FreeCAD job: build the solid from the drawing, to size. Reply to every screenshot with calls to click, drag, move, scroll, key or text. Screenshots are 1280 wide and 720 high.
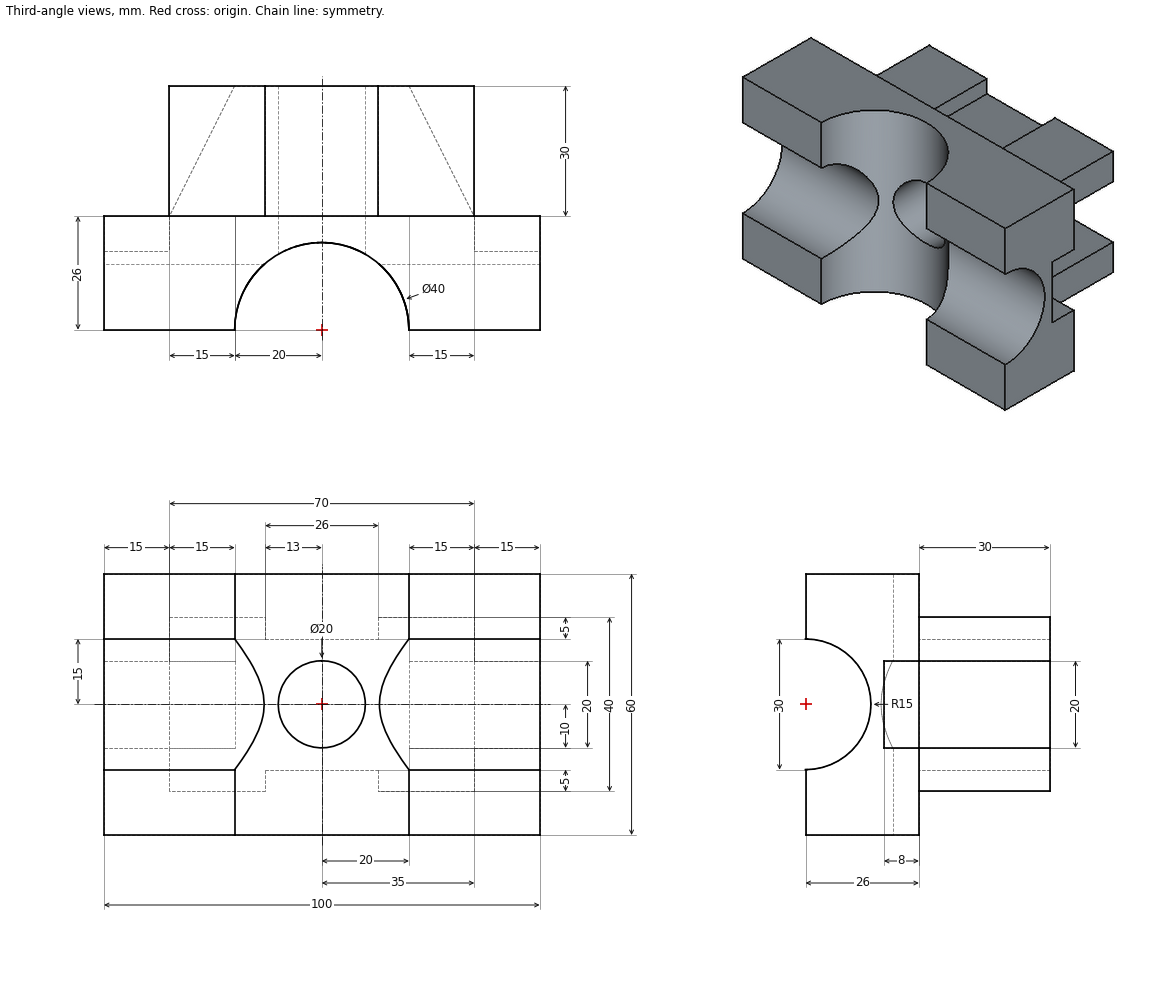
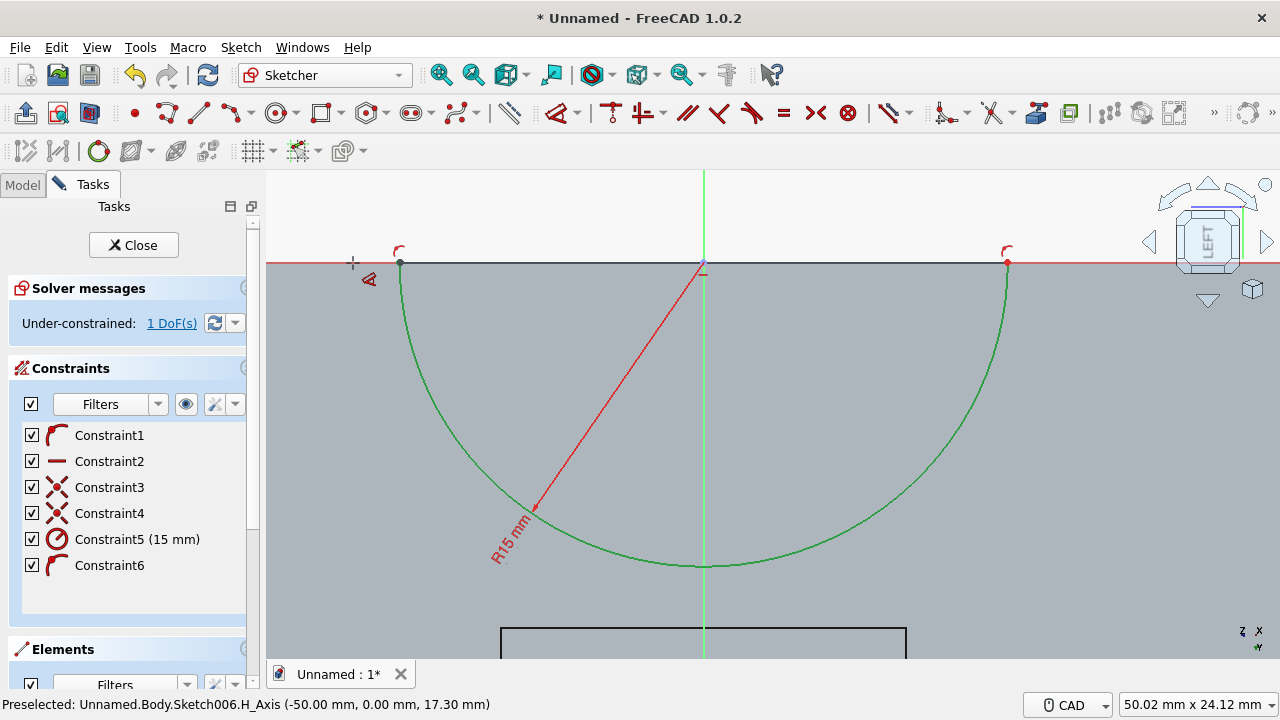
click(825, 263)
click(564, 229)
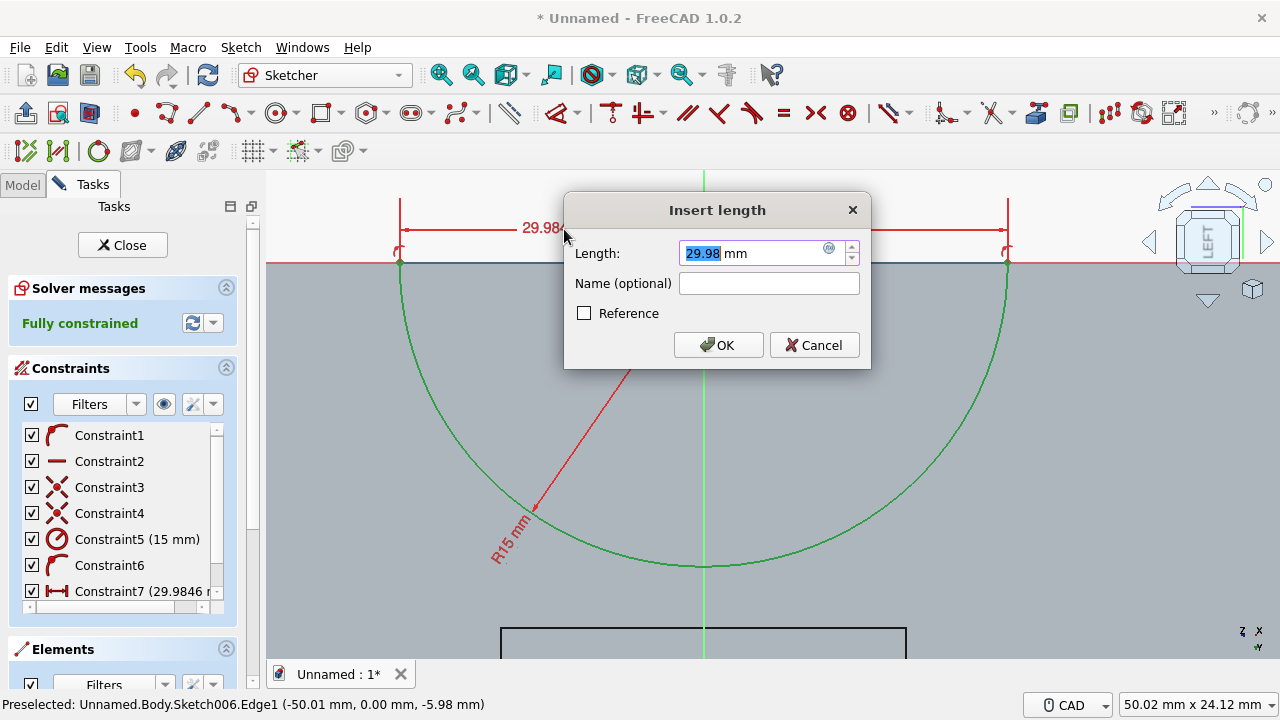
text(30)
key(Return)
key(Escape)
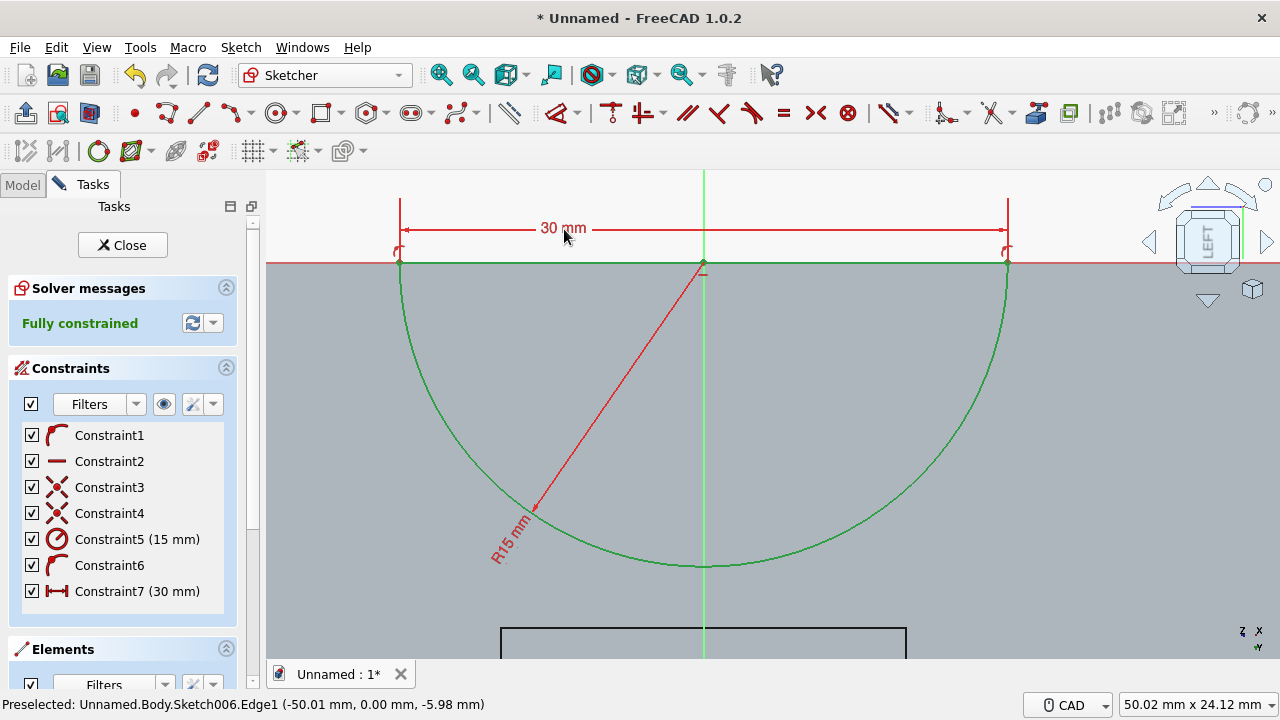
click(123, 245)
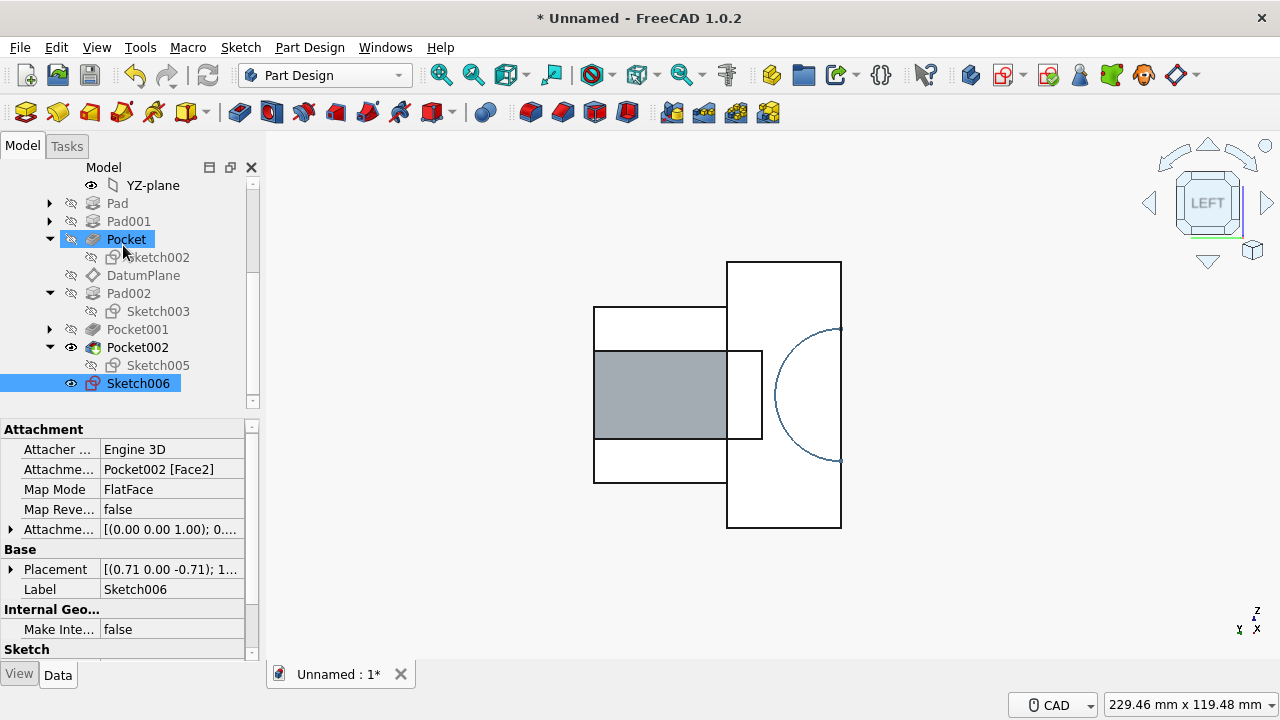
click(240, 112)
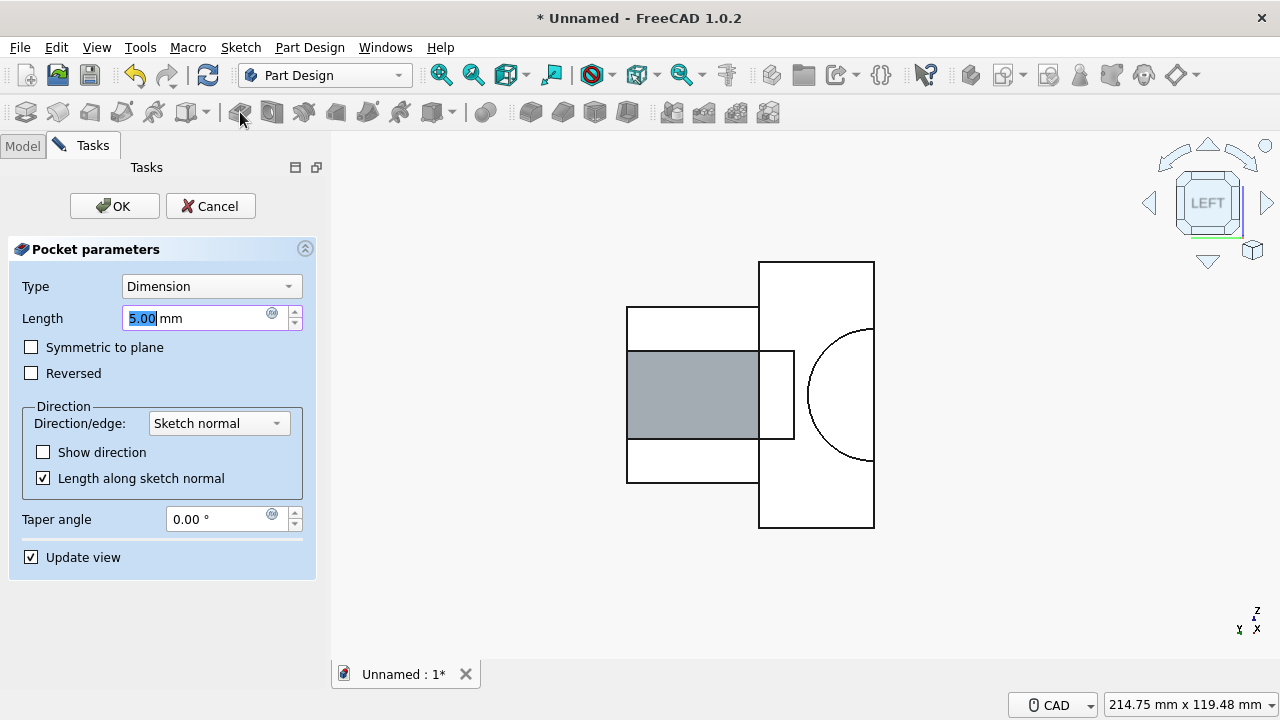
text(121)
key(Tab)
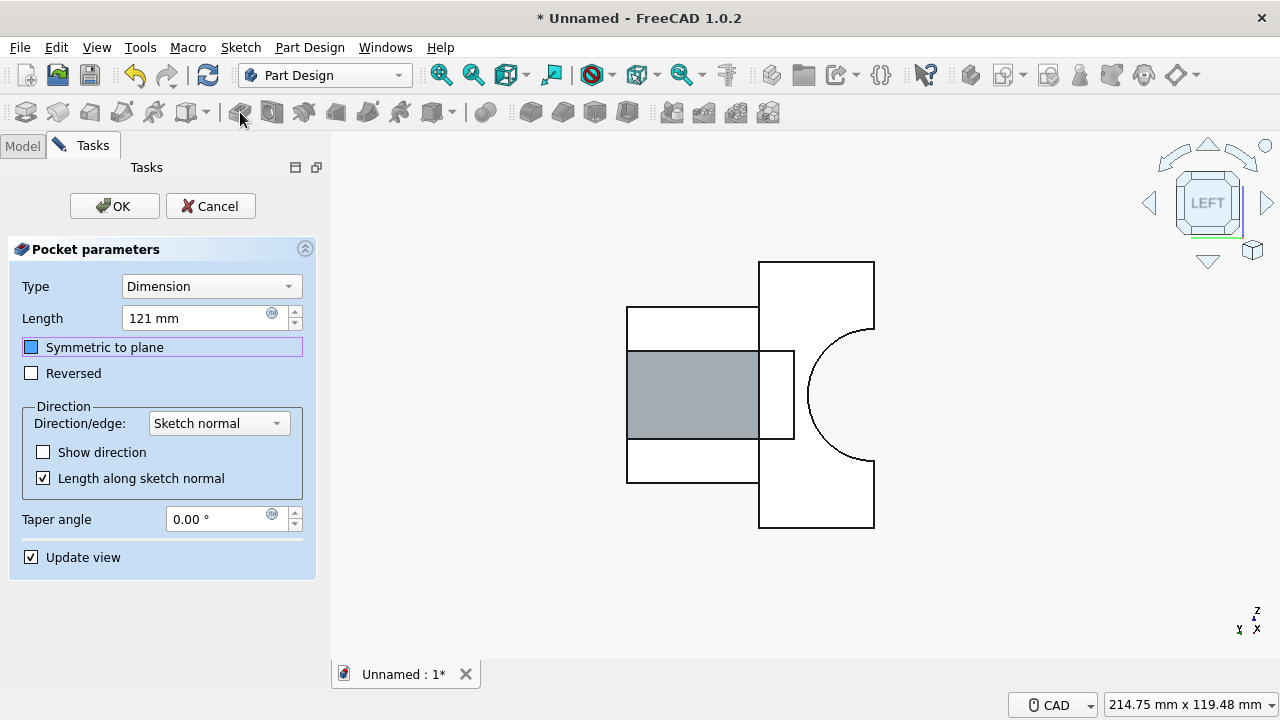
click(115, 206)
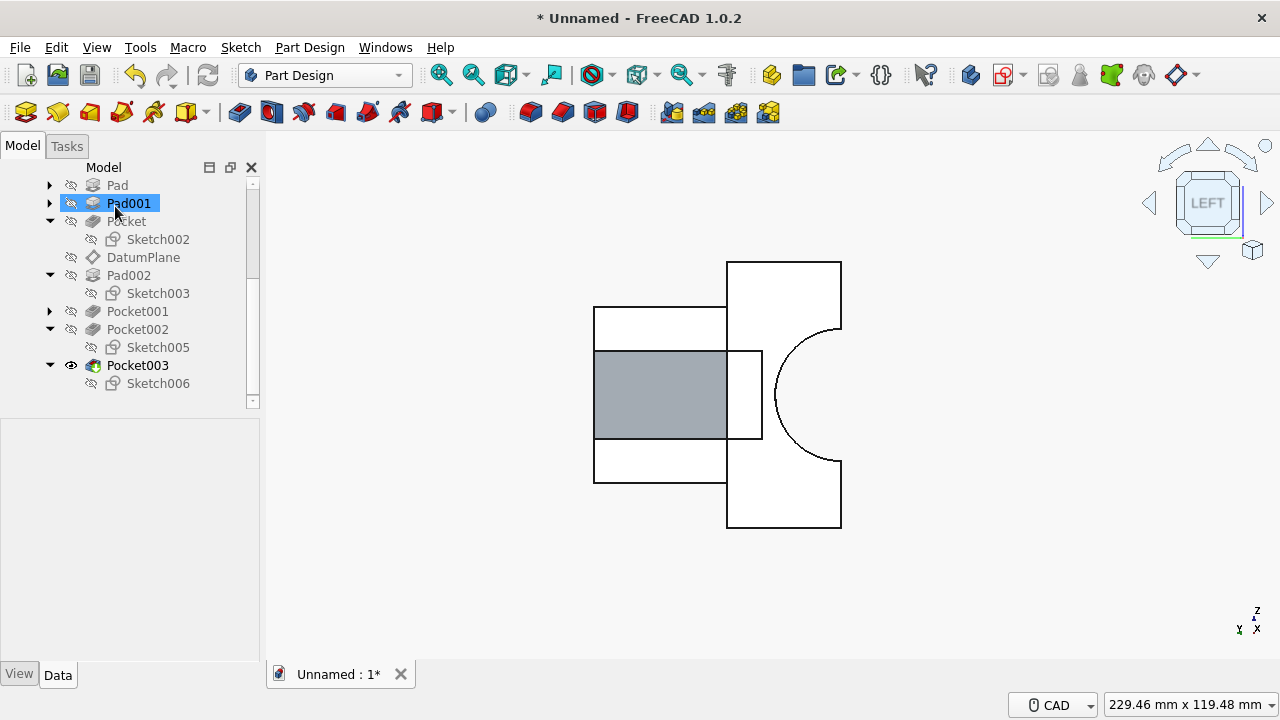
key(5)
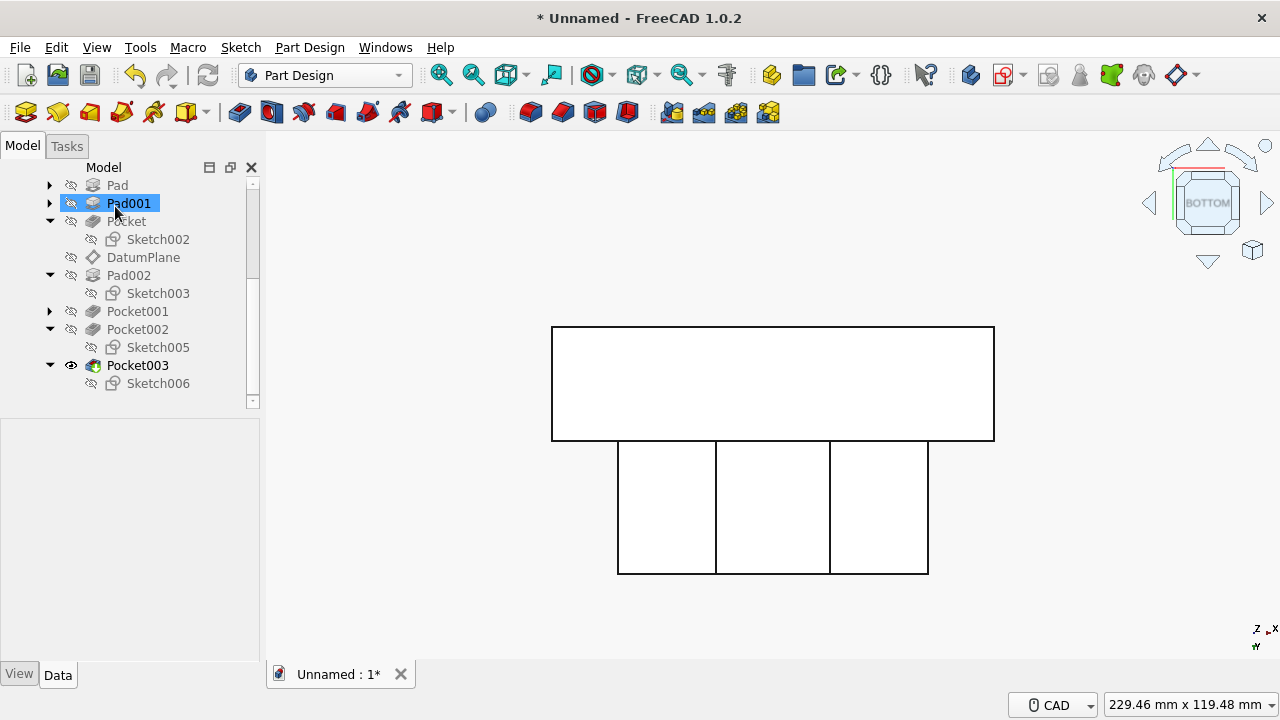
click(899, 383)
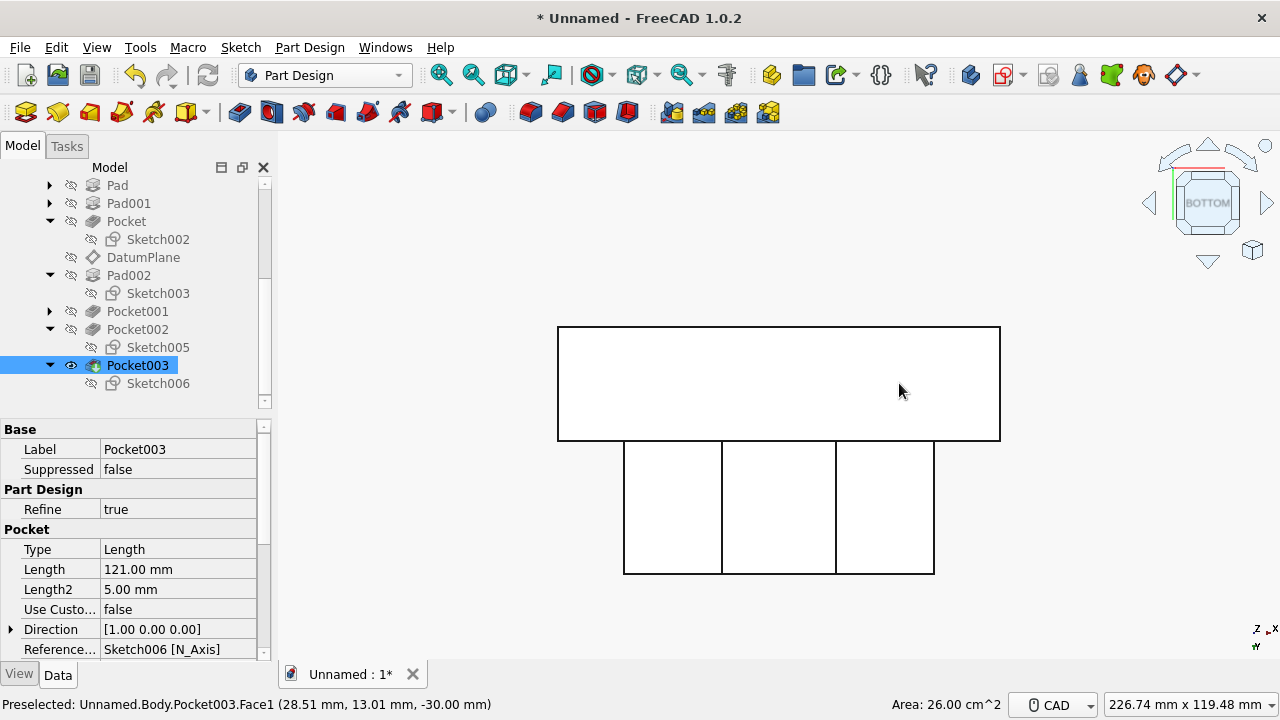
click(1004, 76)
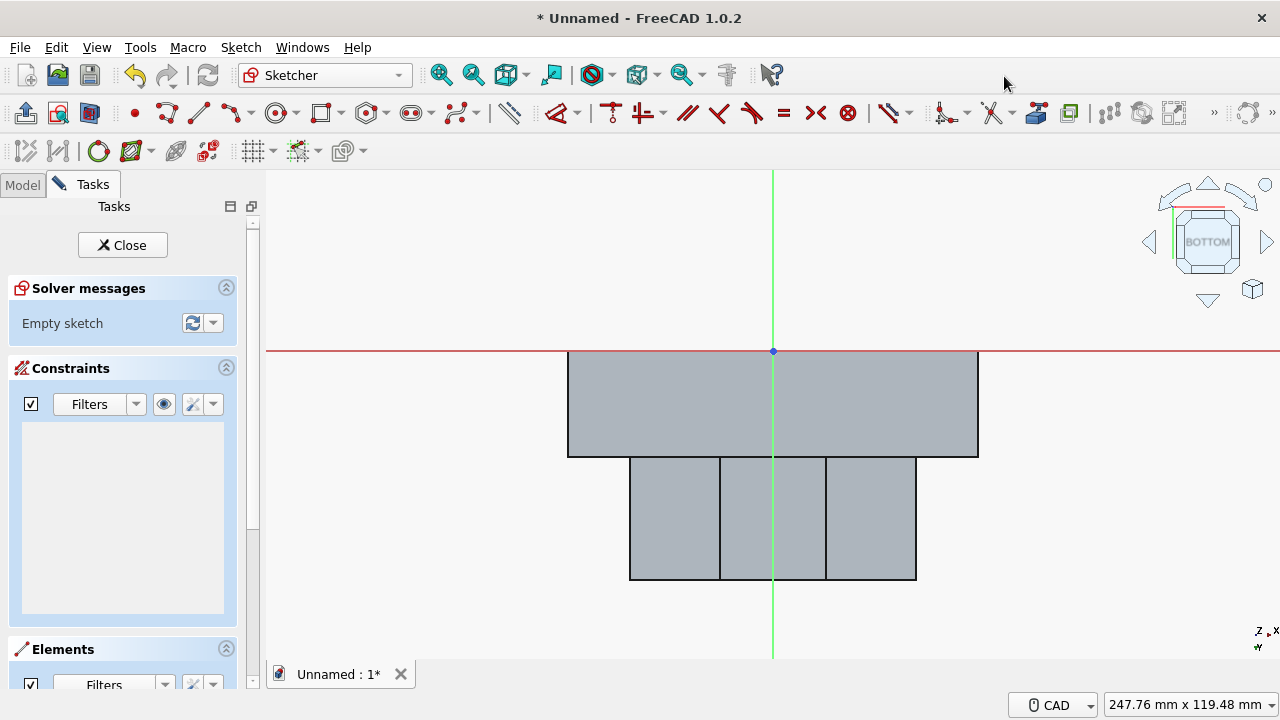
scroll(856, 274, up, 3)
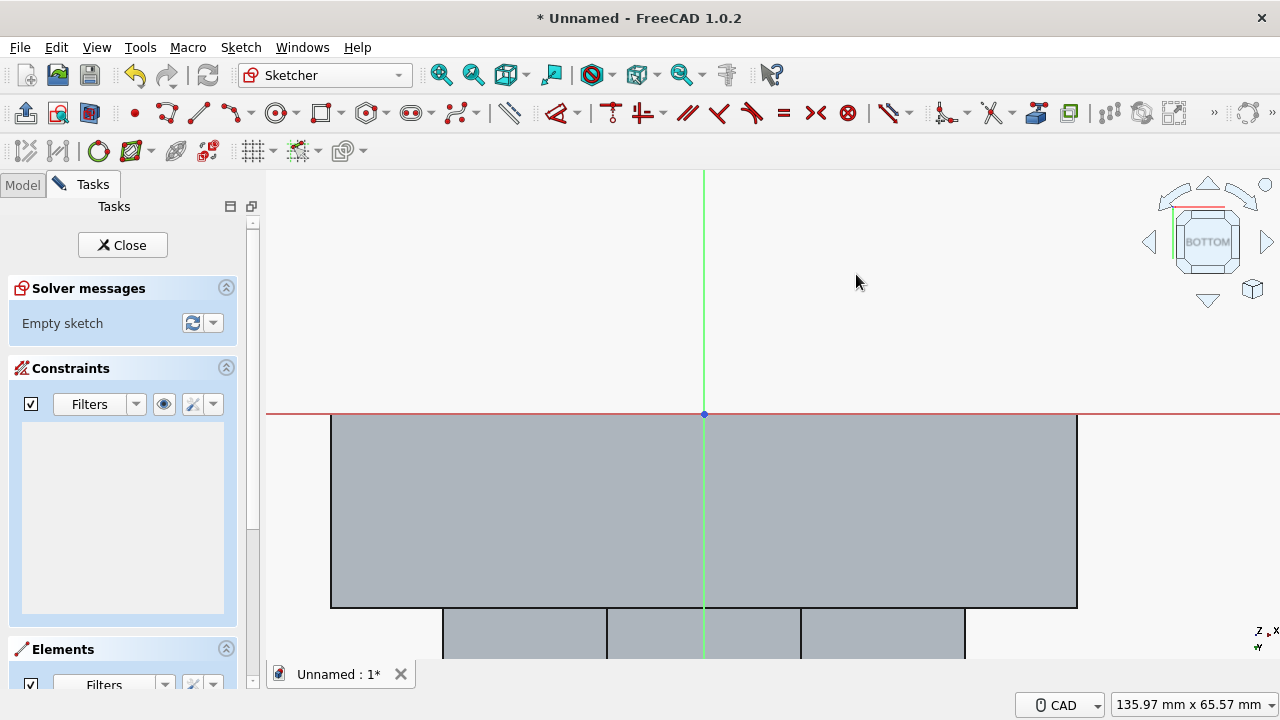
key(g)
key(c)